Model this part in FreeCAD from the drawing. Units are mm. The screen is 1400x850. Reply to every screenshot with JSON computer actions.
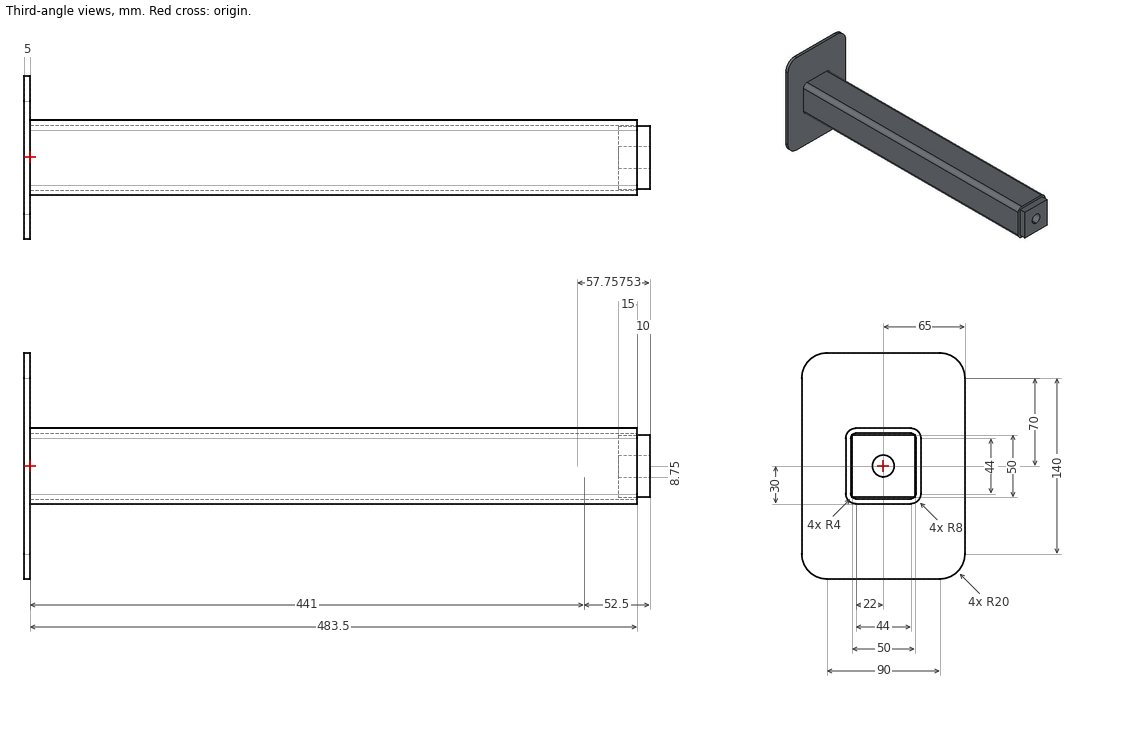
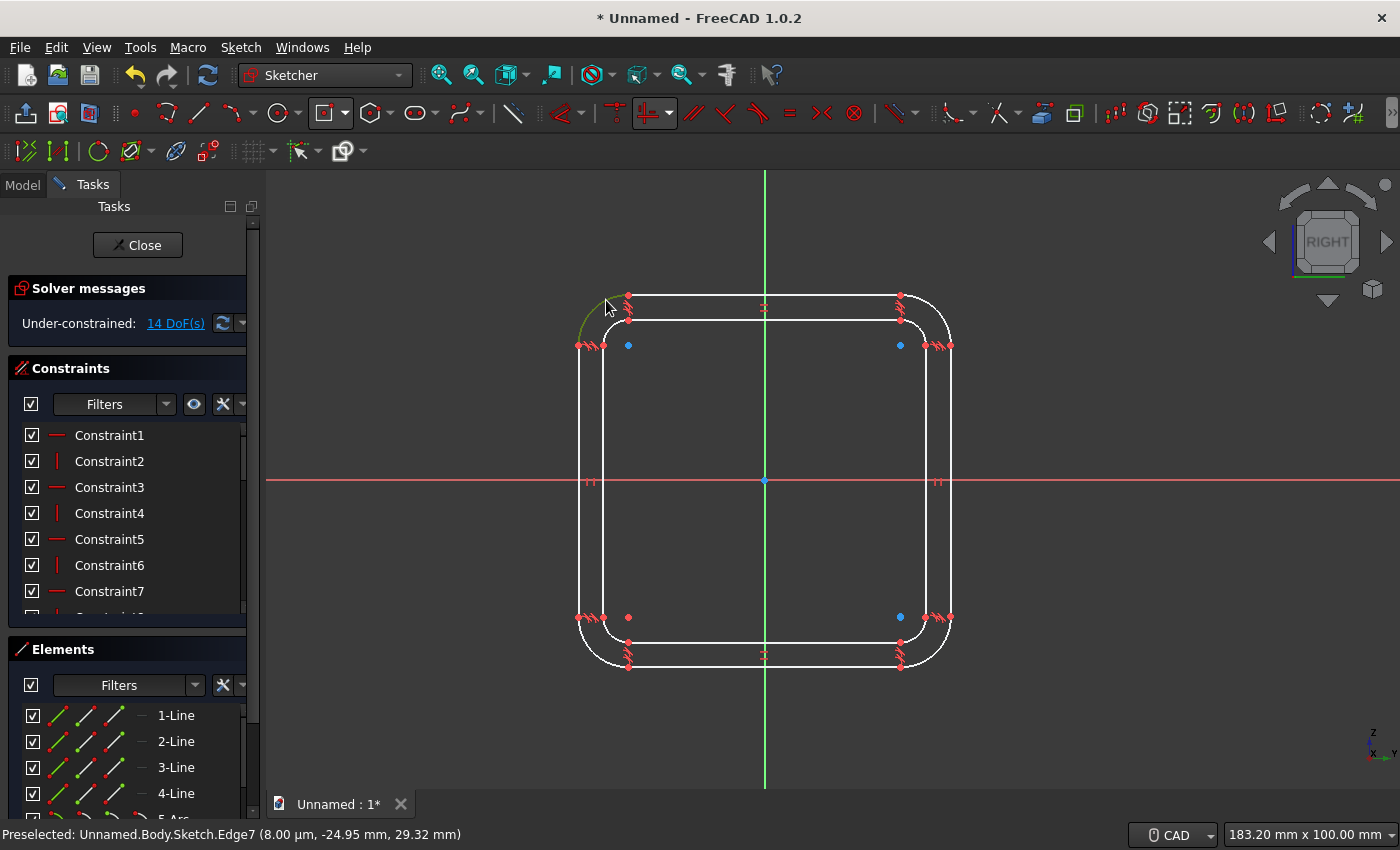
{"action": "left_click", "coordinate": [617, 323]}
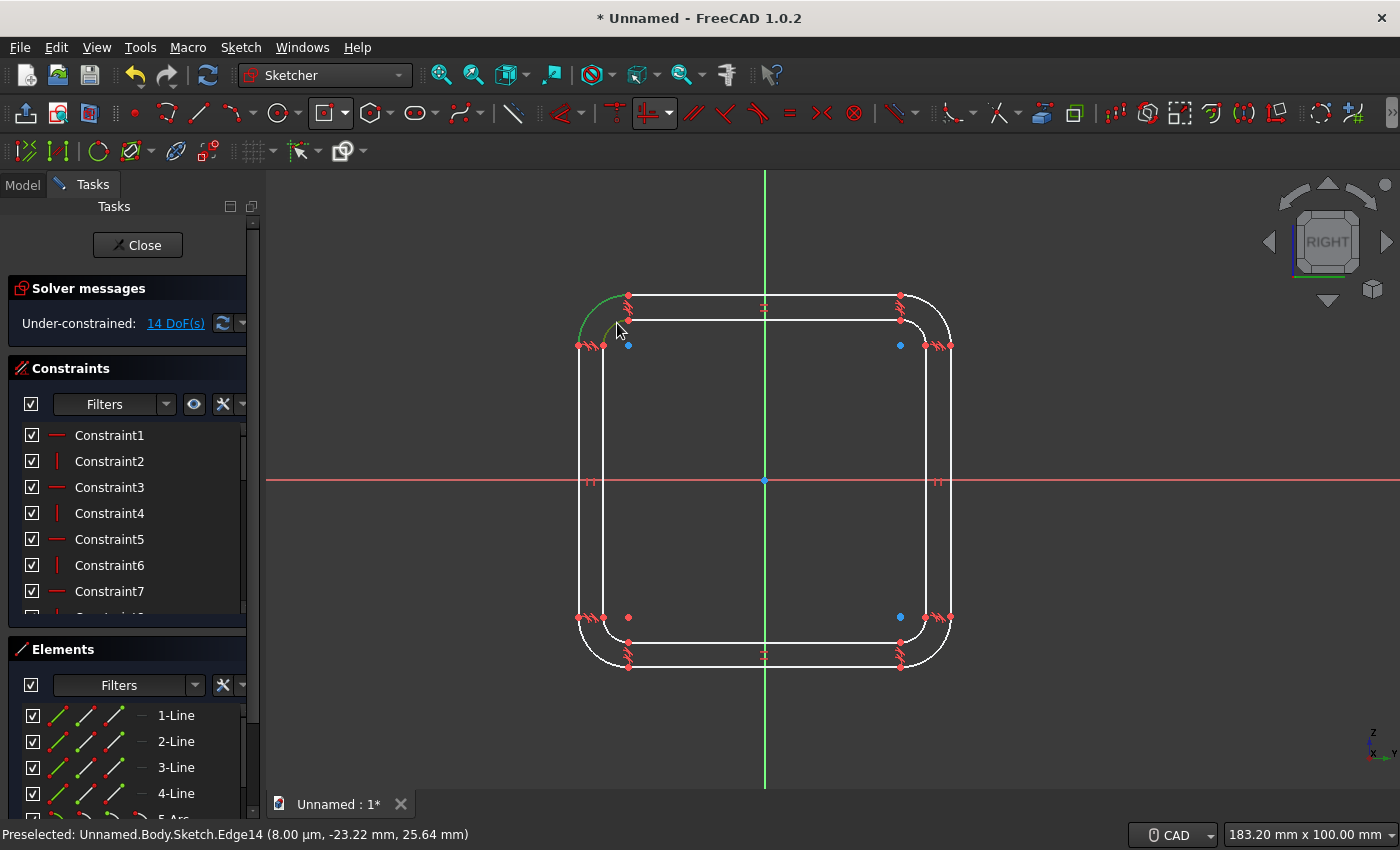
{"action": "left_click", "coordinate": [616, 114]}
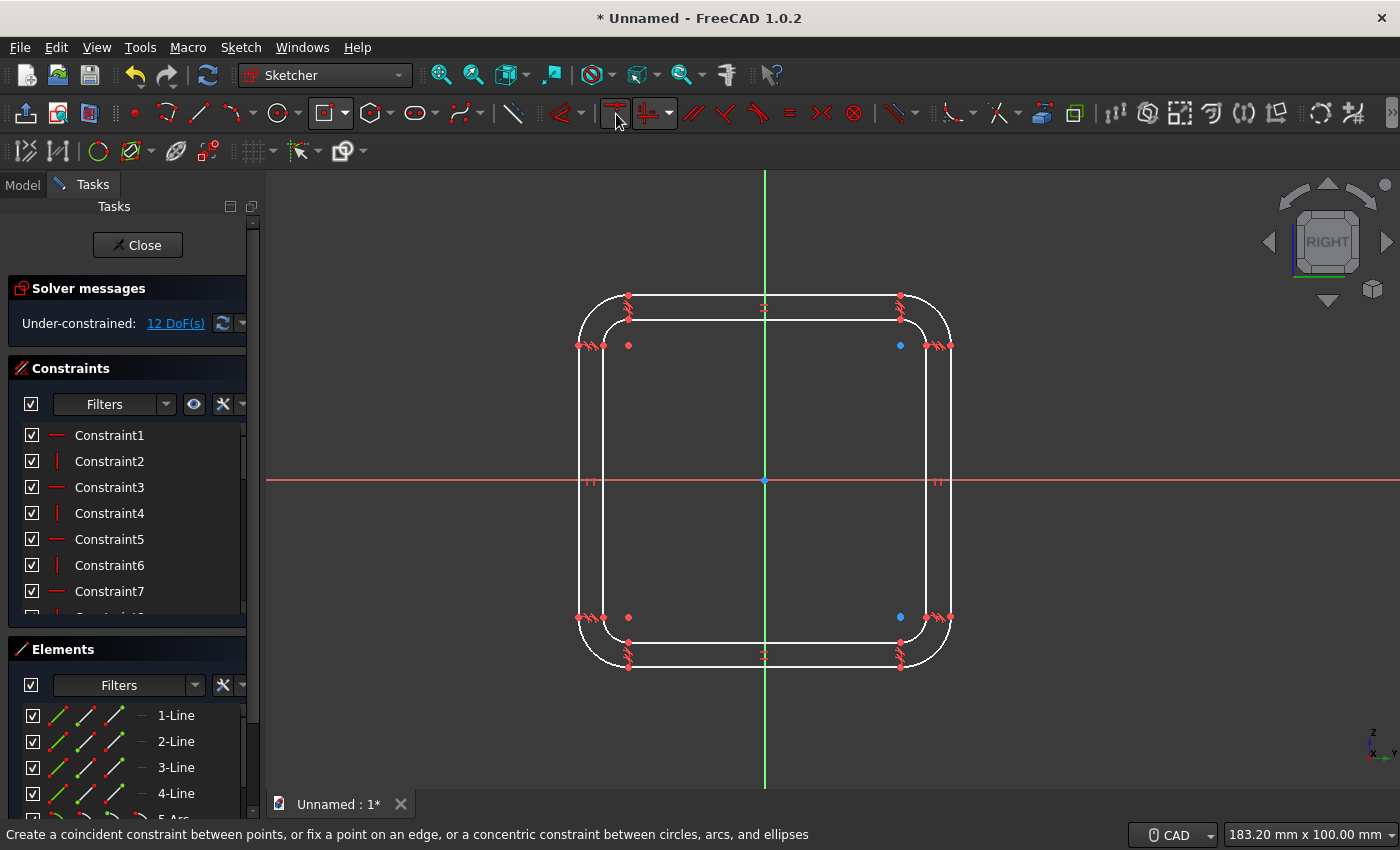
{"action": "left_click", "coordinate": [945, 323]}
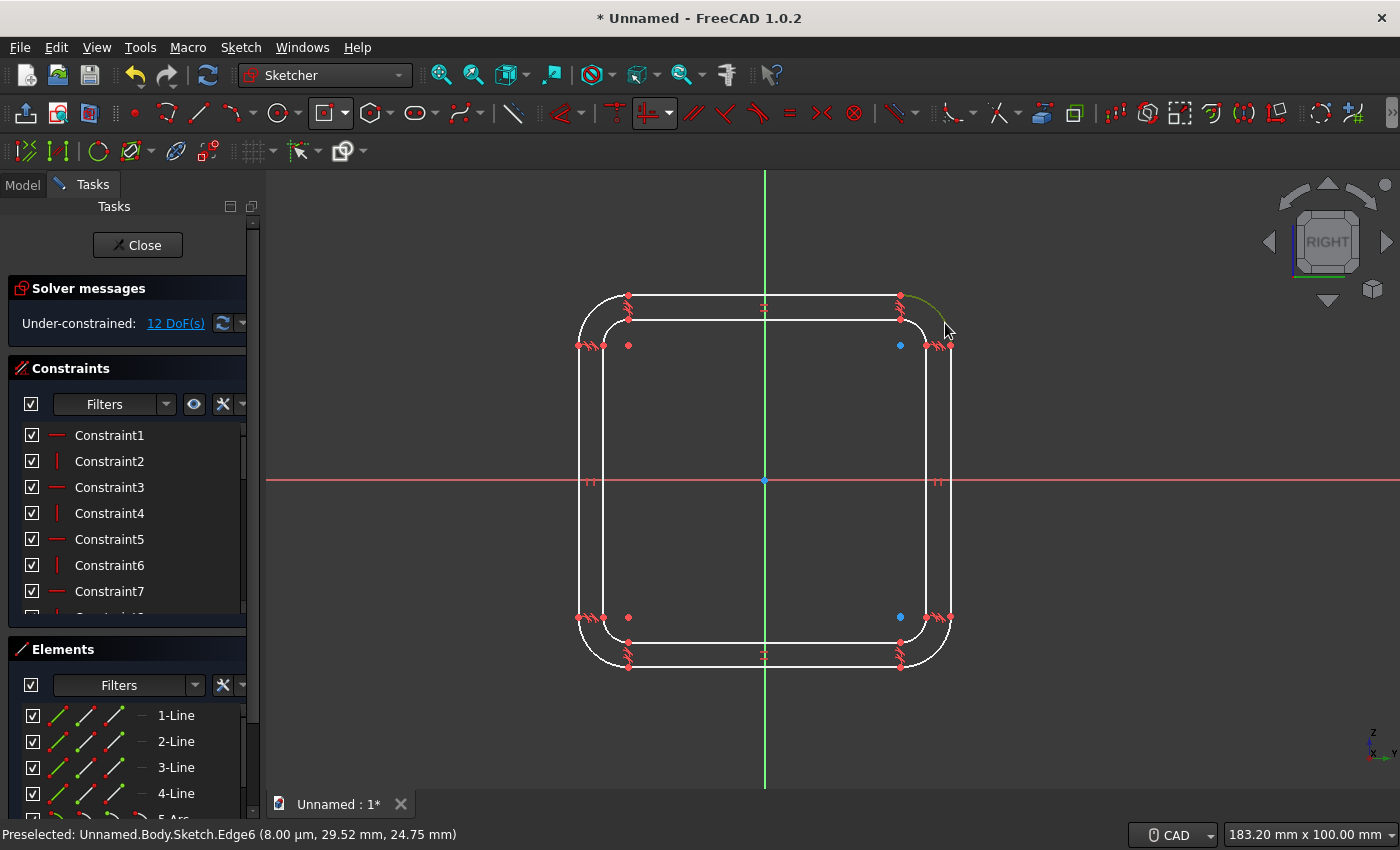
{"action": "left_click", "coordinate": [923, 334]}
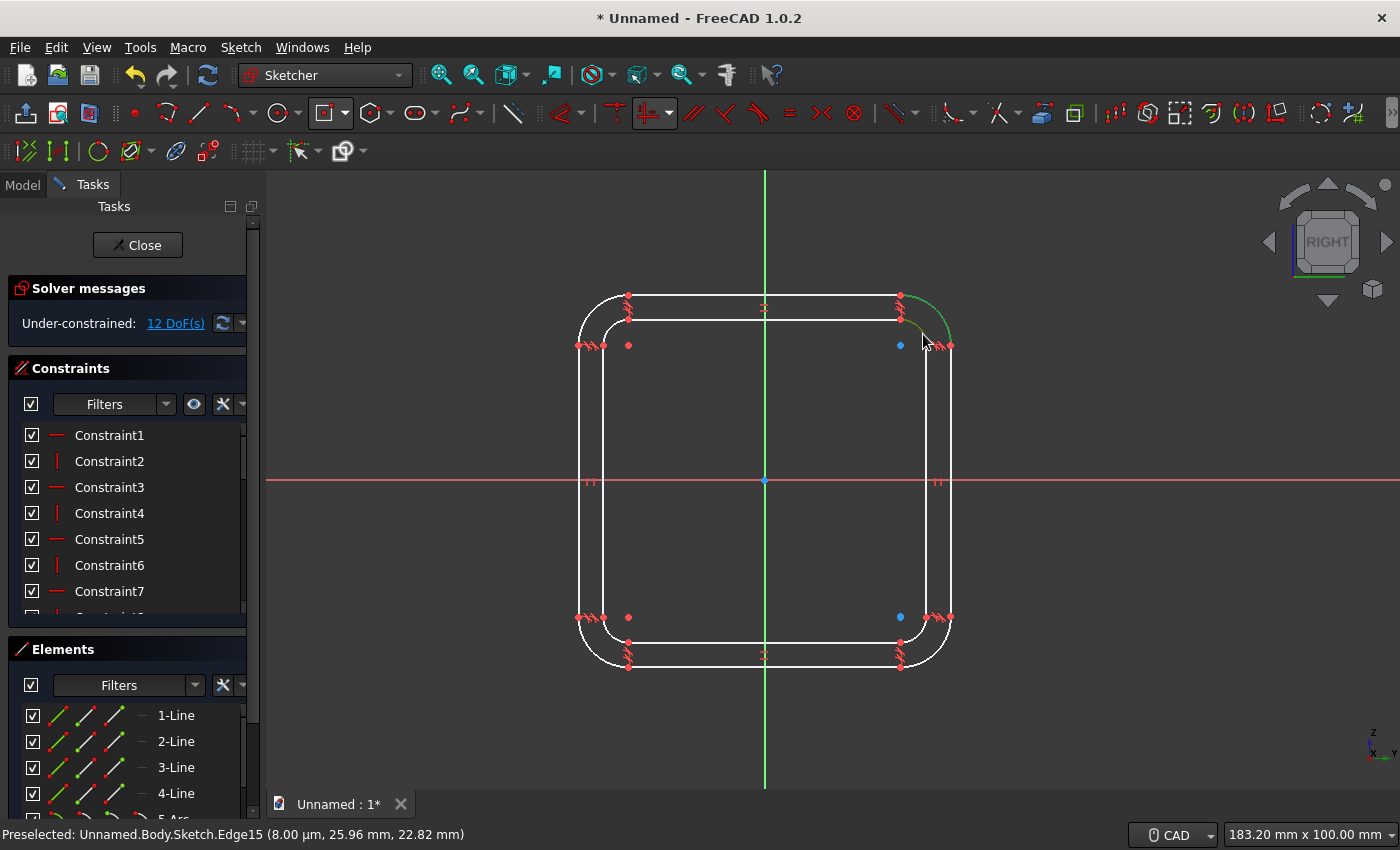
{"action": "left_click", "coordinate": [616, 114]}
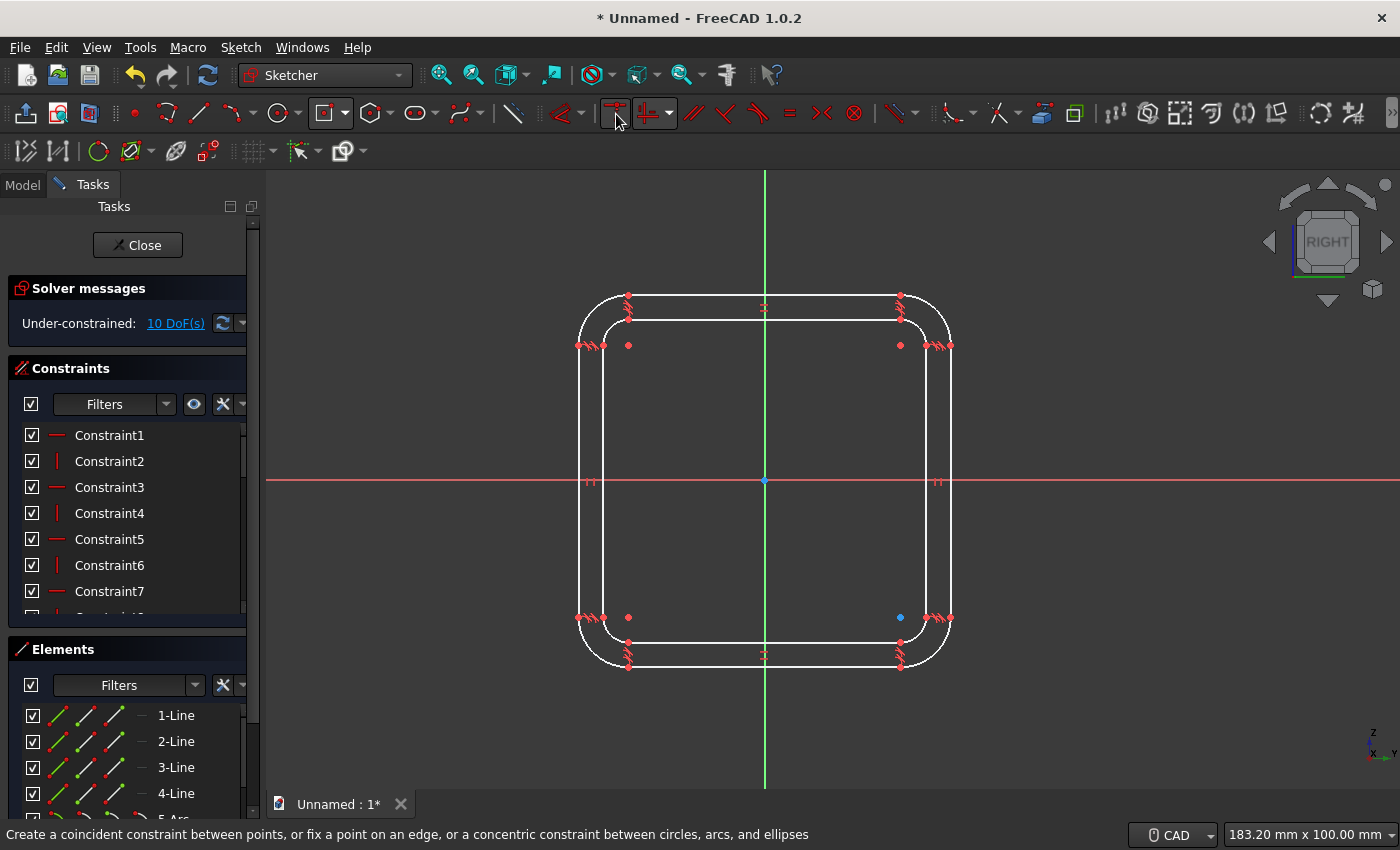
{"action": "left_click", "coordinate": [923, 662]}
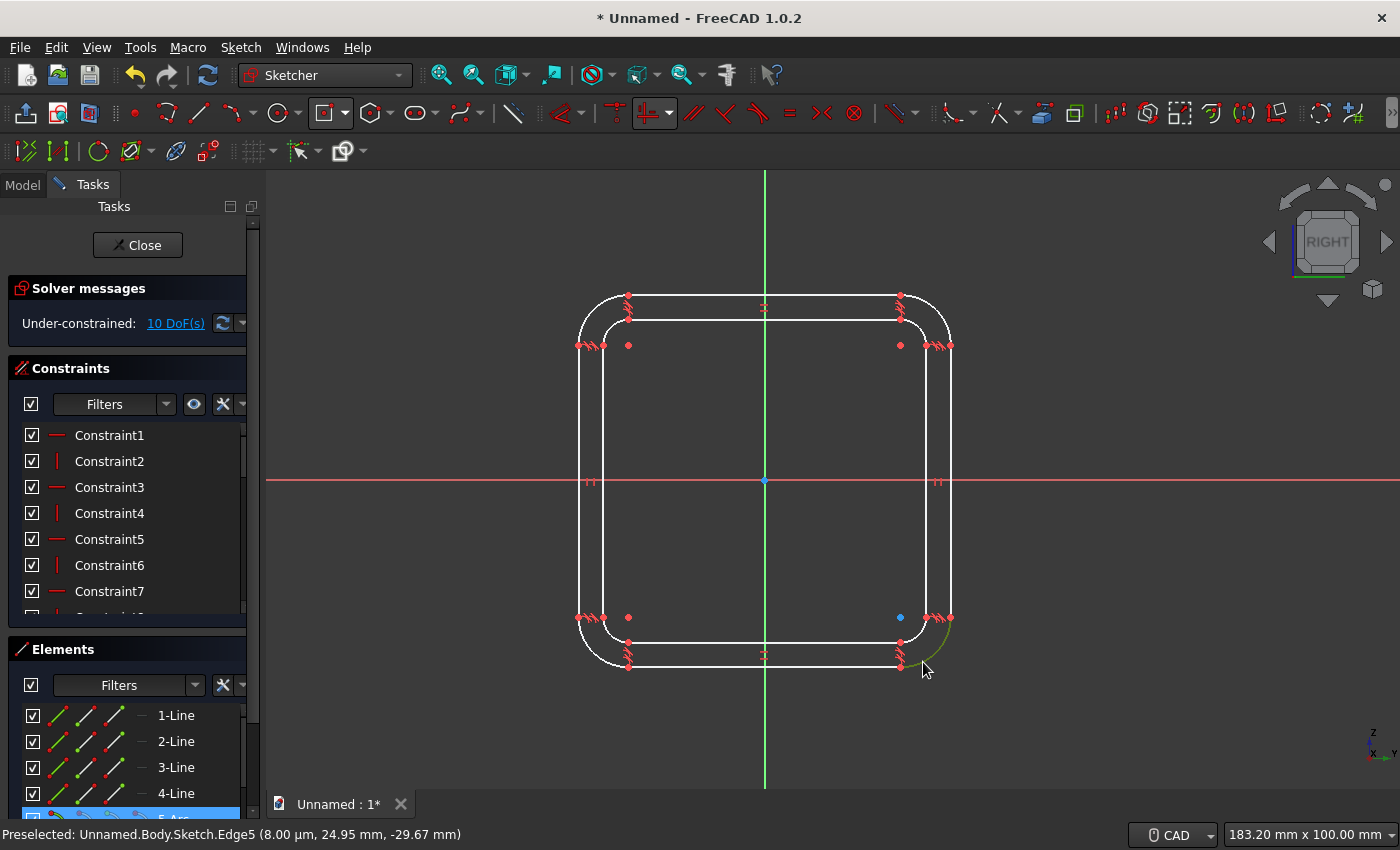
{"action": "left_click", "coordinate": [945, 322]}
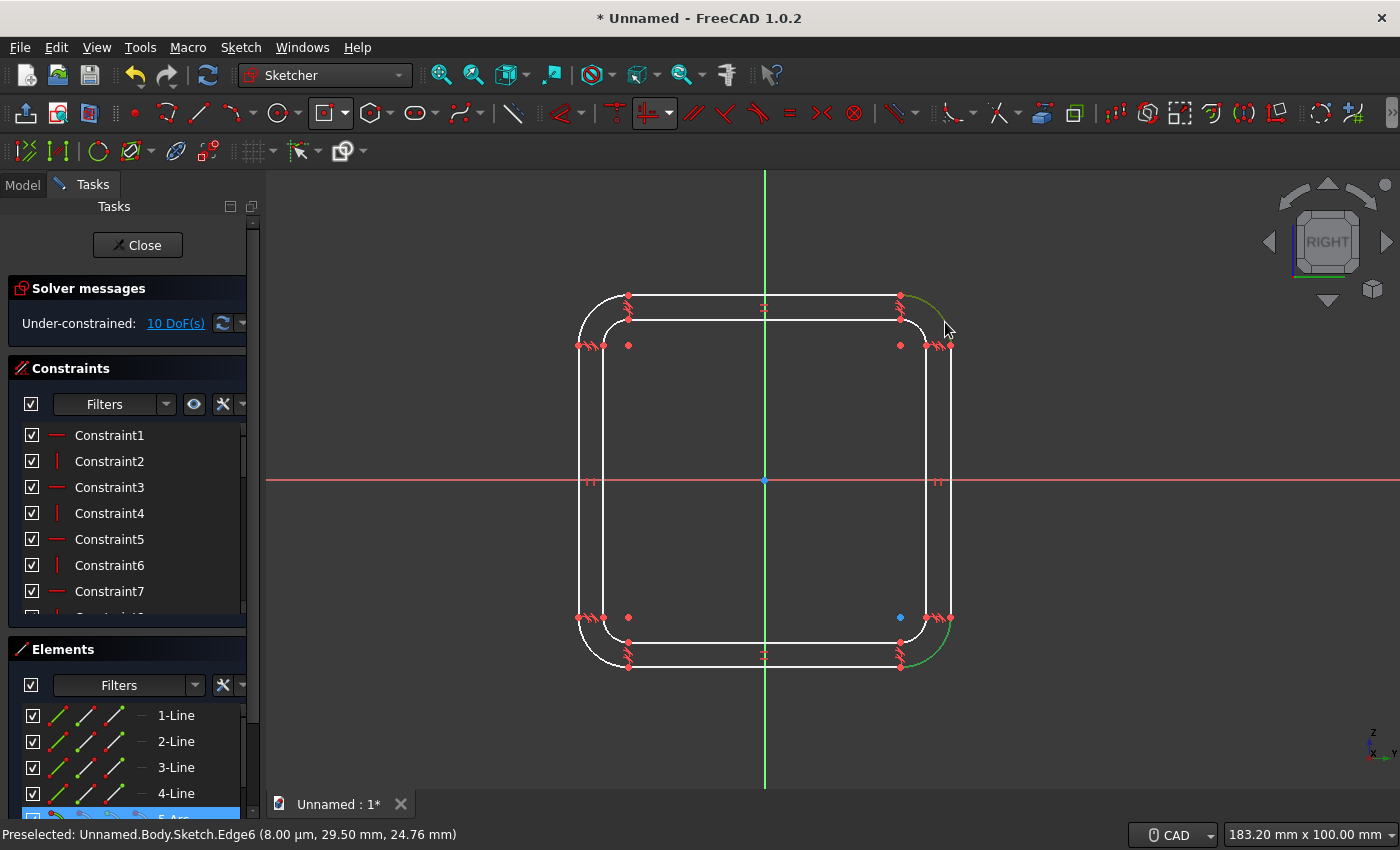
{"action": "left_click", "coordinate": [606, 301]}